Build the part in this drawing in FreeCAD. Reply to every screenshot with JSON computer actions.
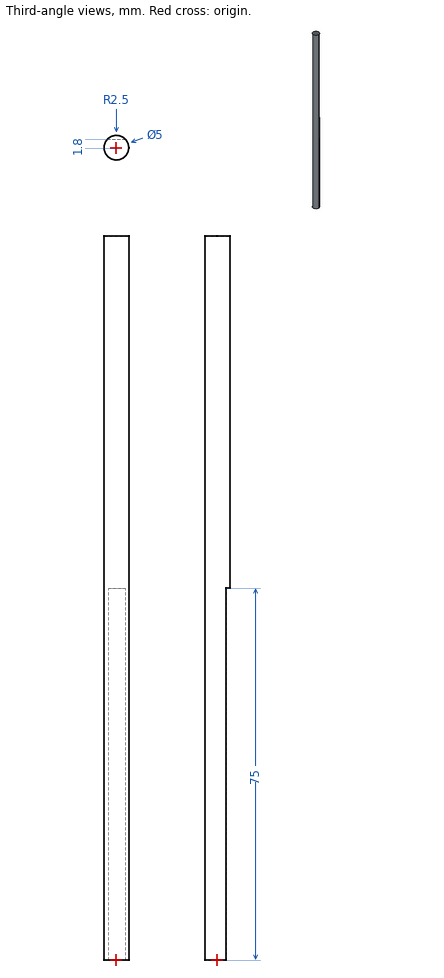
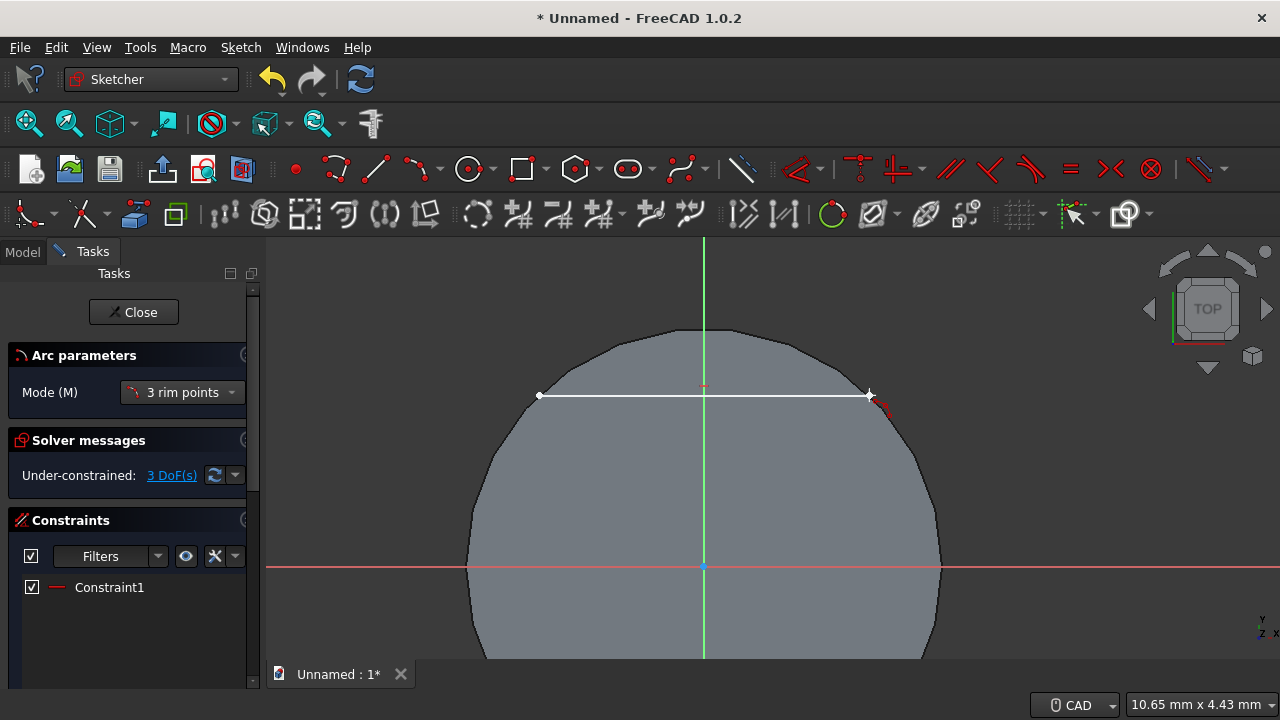
{"action": "left_click", "coordinate": [869, 396]}
{"action": "left_click", "coordinate": [539, 396]}
{"action": "left_click", "coordinate": [740, 332]}
{"action": "key", "text": "Escape"}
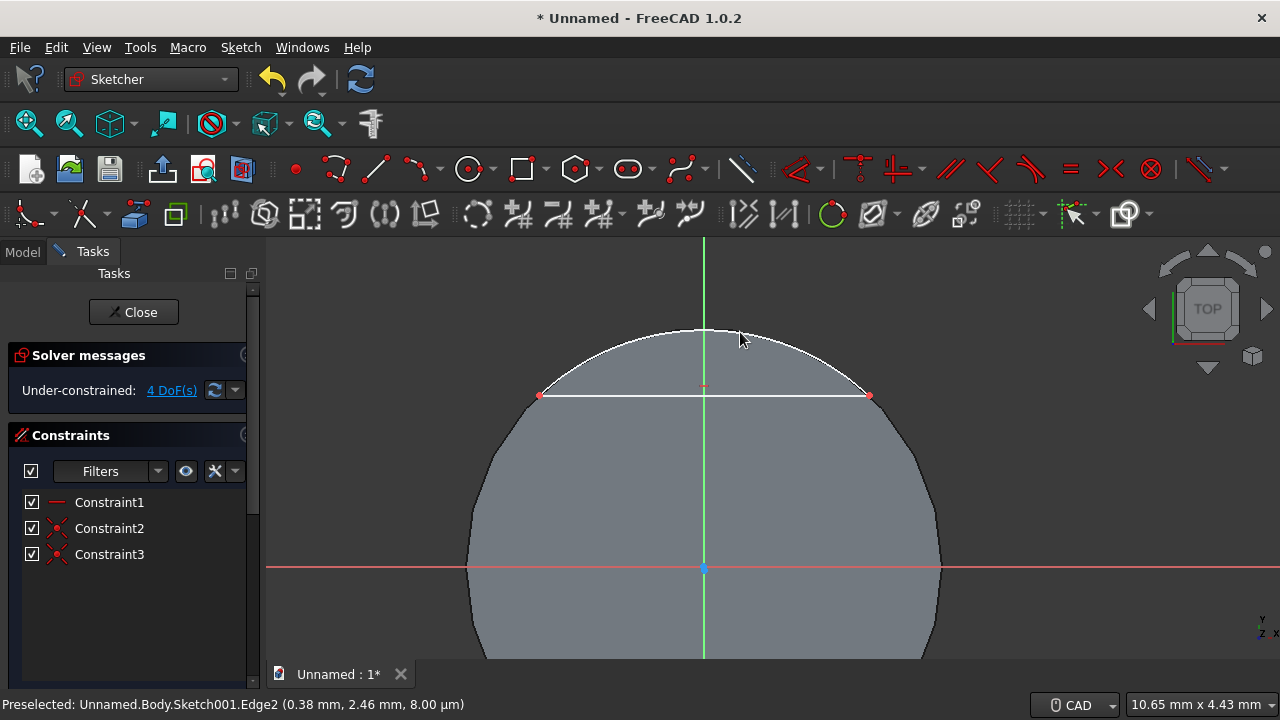
{"action": "left_click_drag", "start_coordinate": [694, 557], "coordinate": [714, 580]}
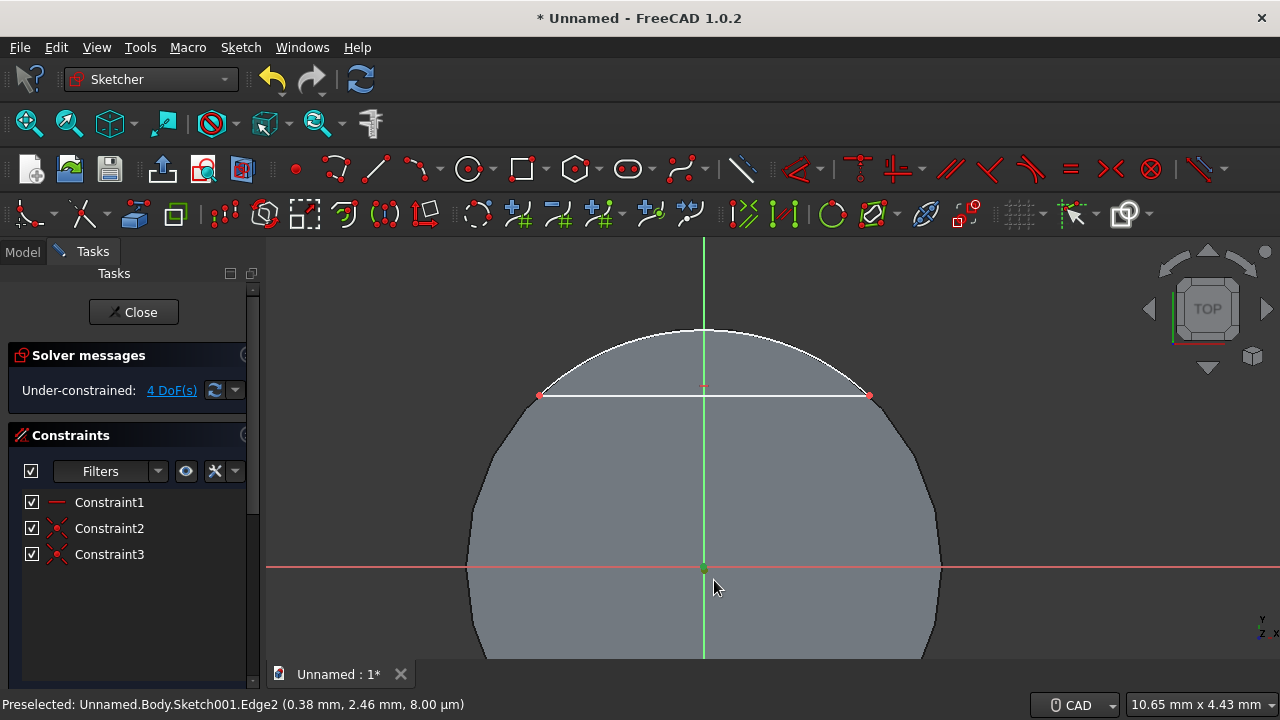
{"action": "left_click", "coordinate": [858, 170]}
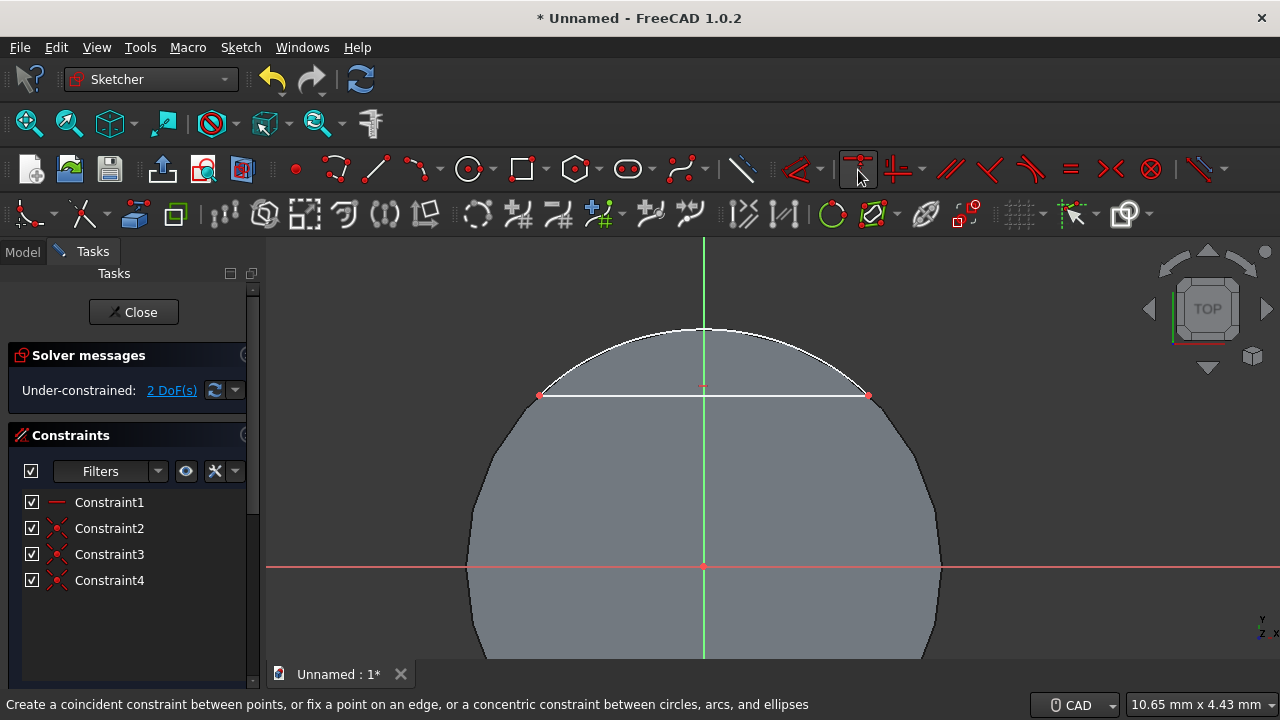
{"action": "left_click", "coordinate": [776, 340]}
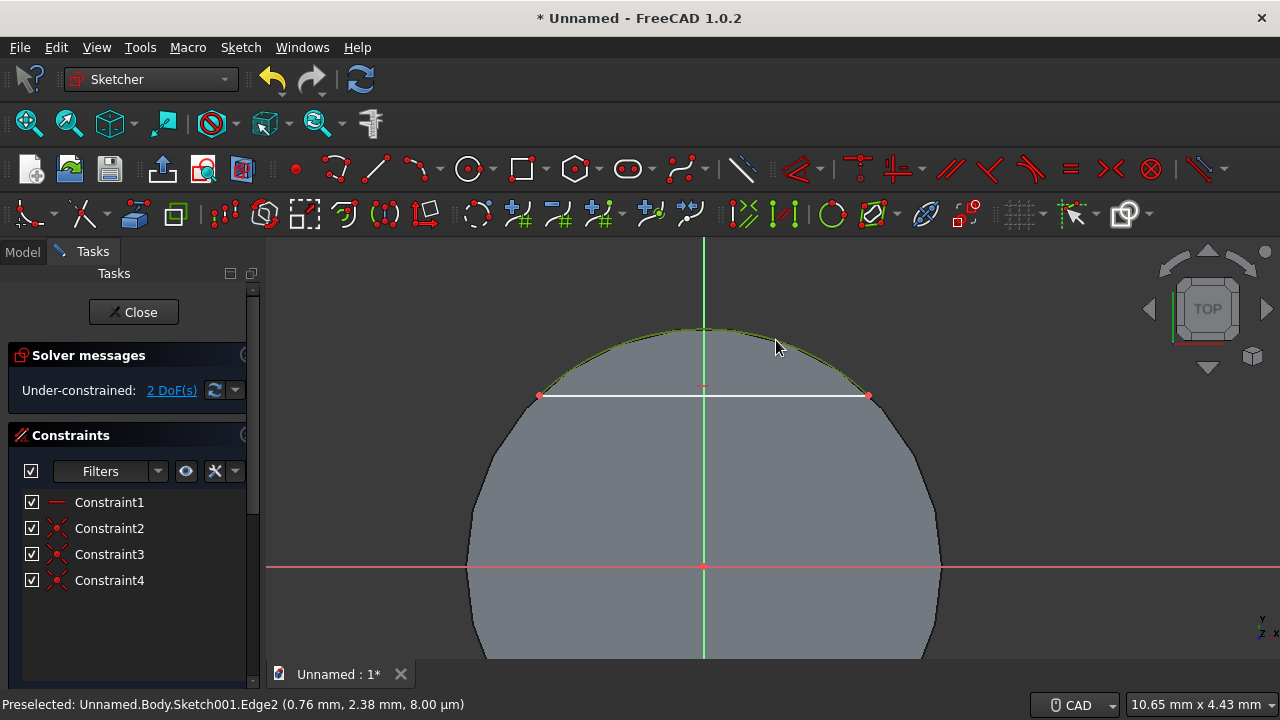
{"action": "left_click", "coordinate": [822, 170]}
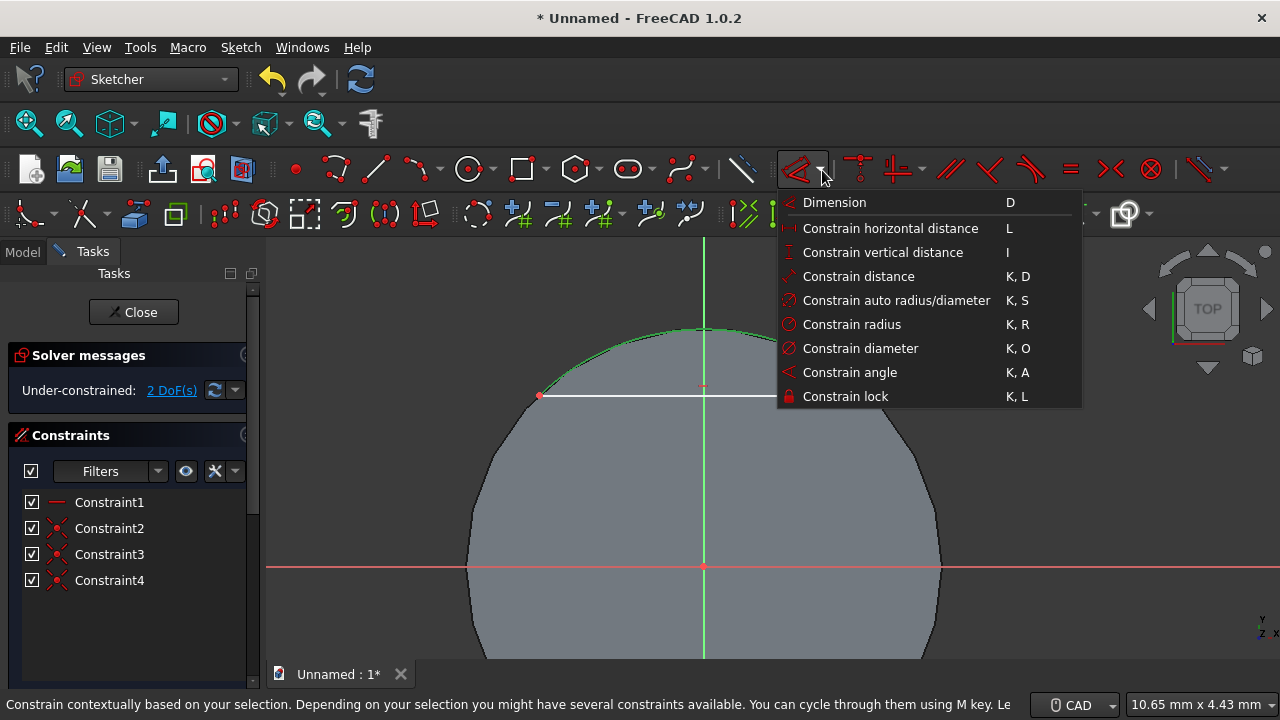
{"action": "left_click", "coordinate": [930, 324]}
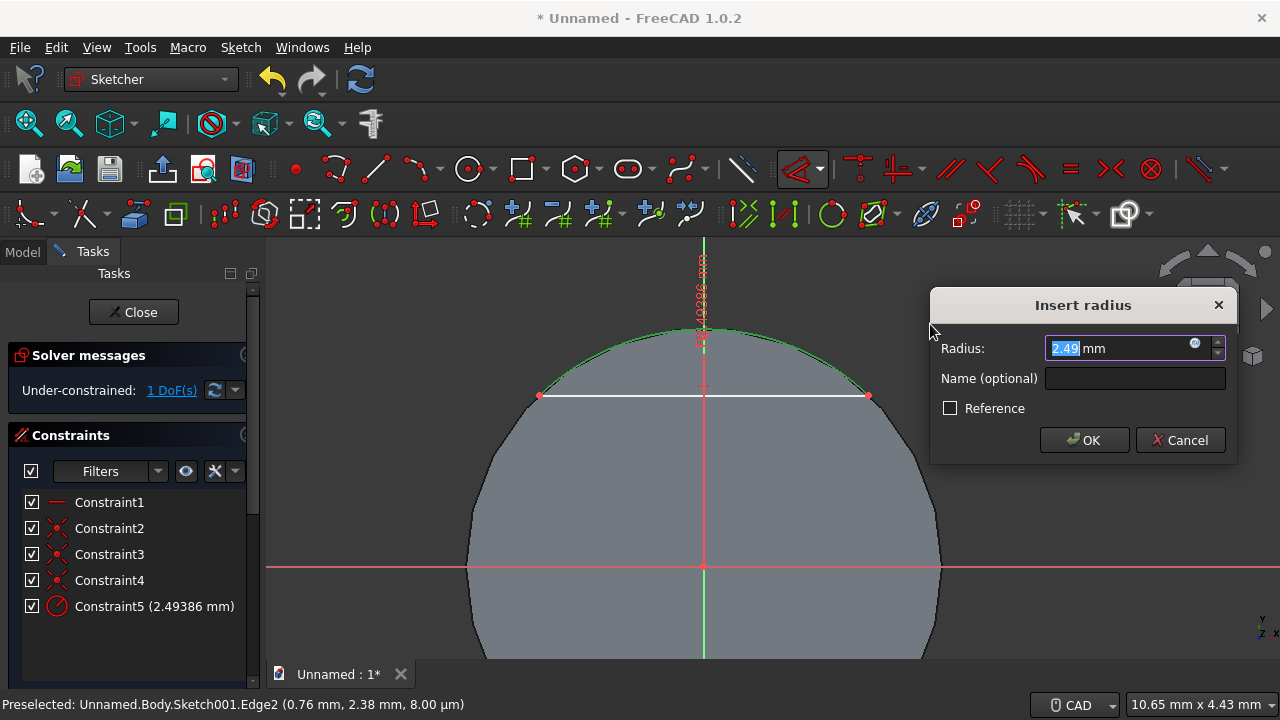
{"action": "type", "text": "2.5"}
{"action": "key", "text": "Return"}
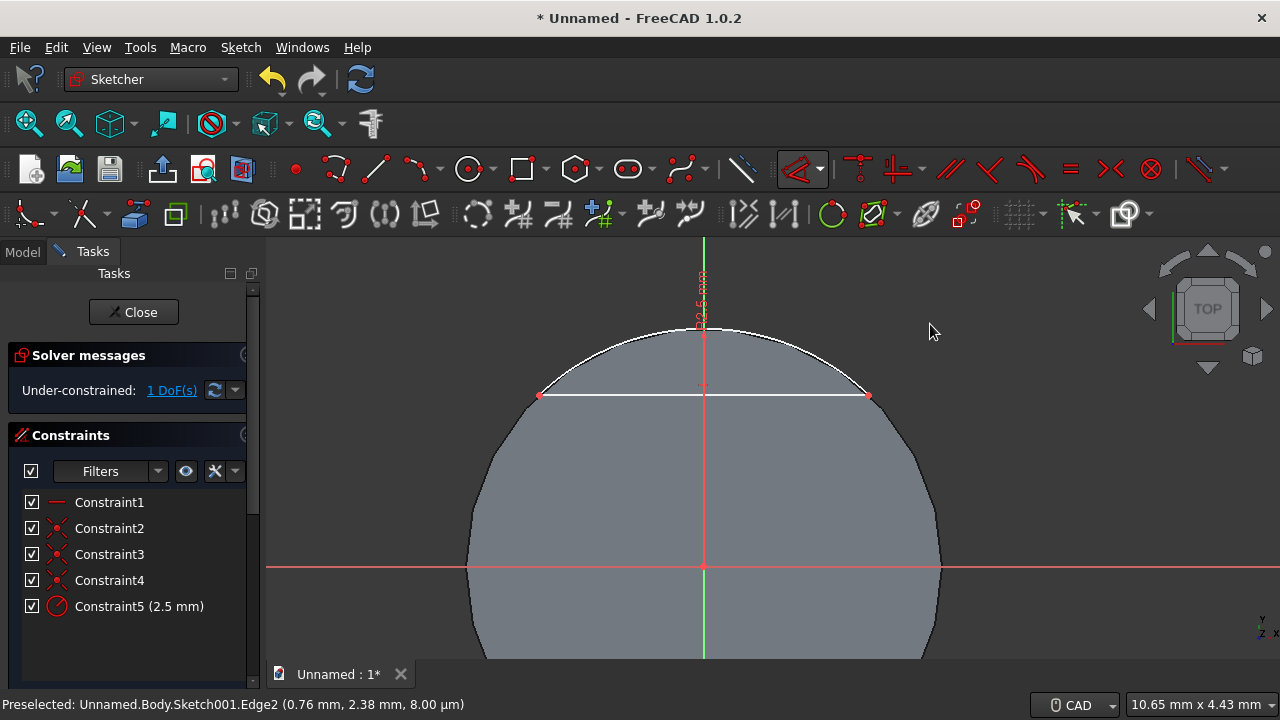
{"action": "left_click", "coordinate": [539, 395]}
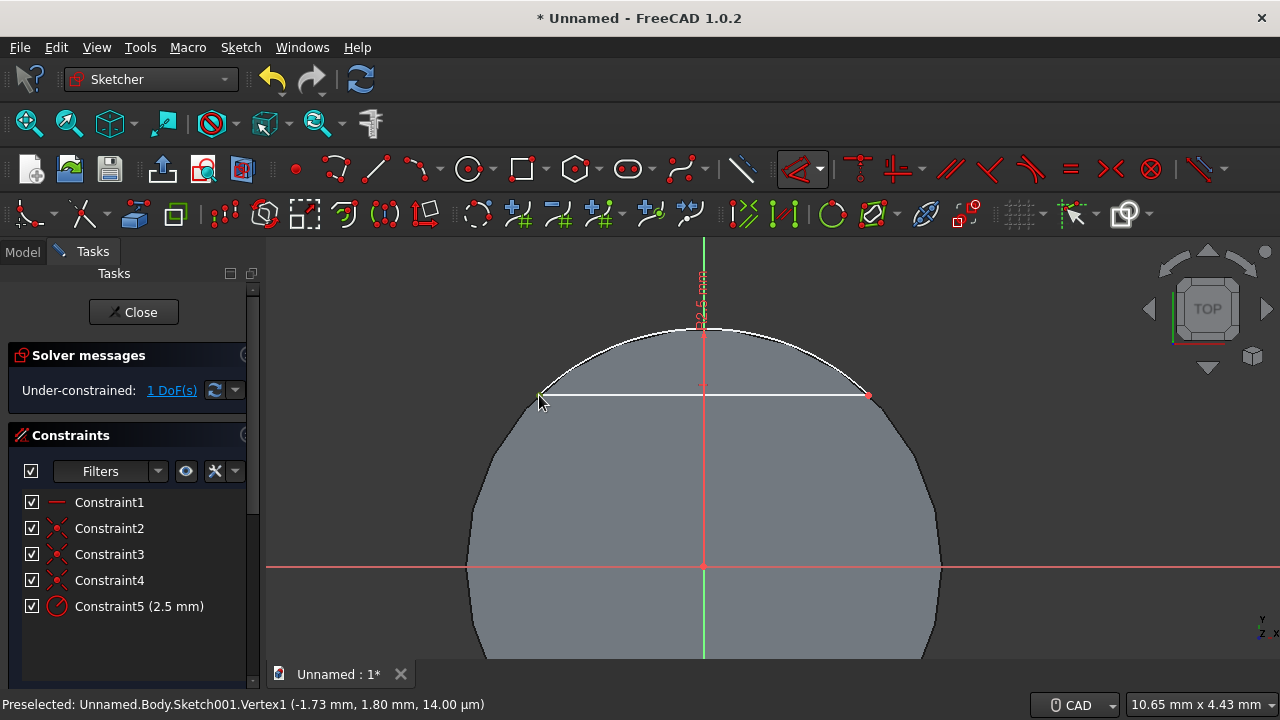
{"action": "key", "text": "i"}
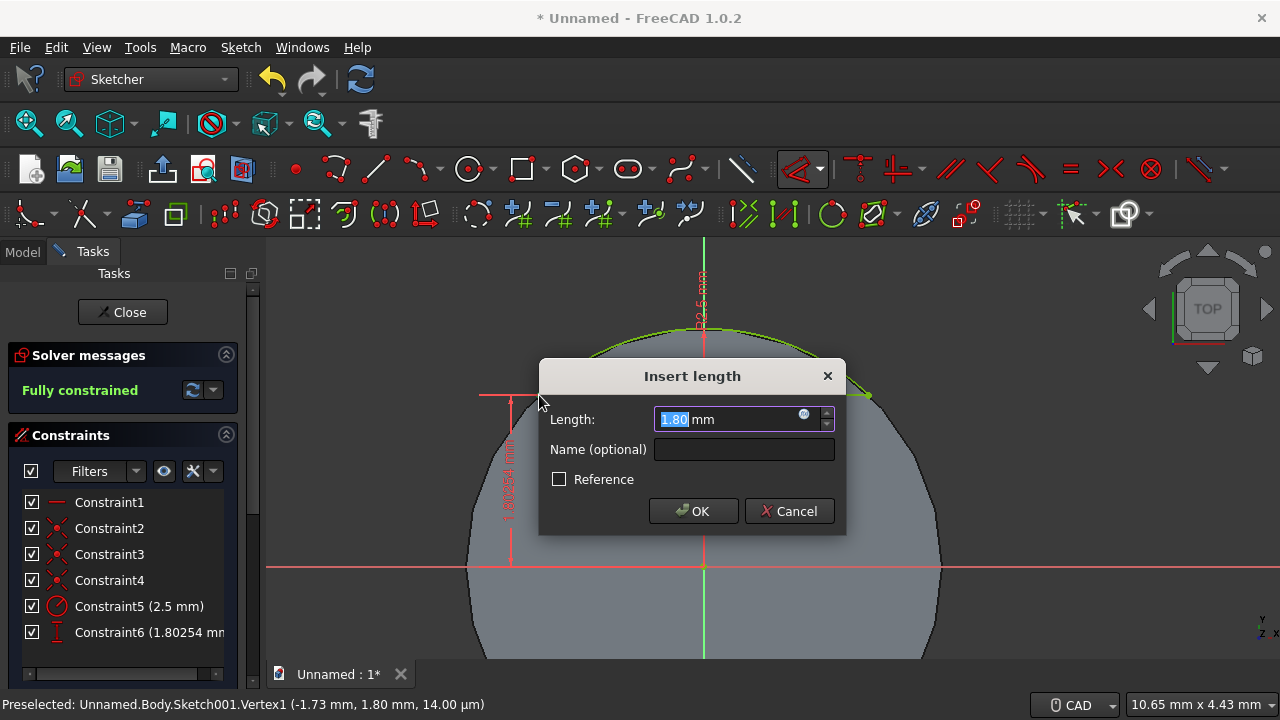
{"action": "type", "text": "1.8"}
{"action": "key", "text": "Return"}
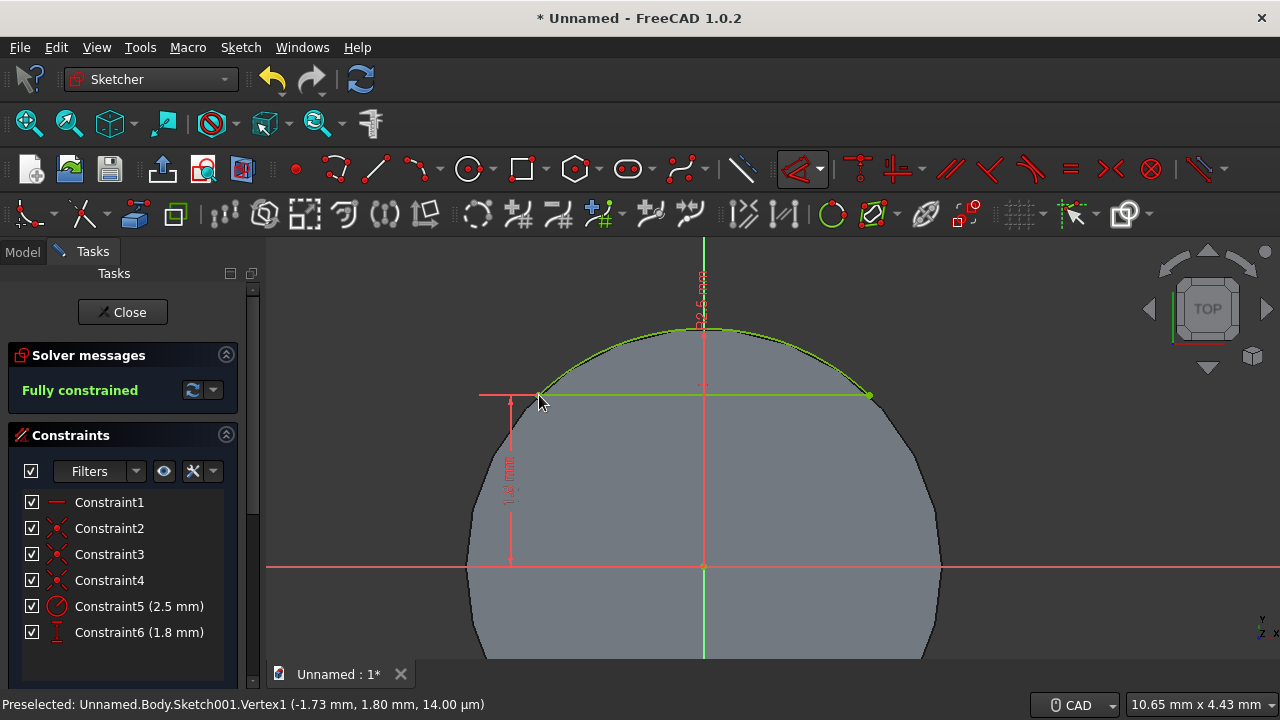
{"action": "left_click", "coordinate": [123, 312]}